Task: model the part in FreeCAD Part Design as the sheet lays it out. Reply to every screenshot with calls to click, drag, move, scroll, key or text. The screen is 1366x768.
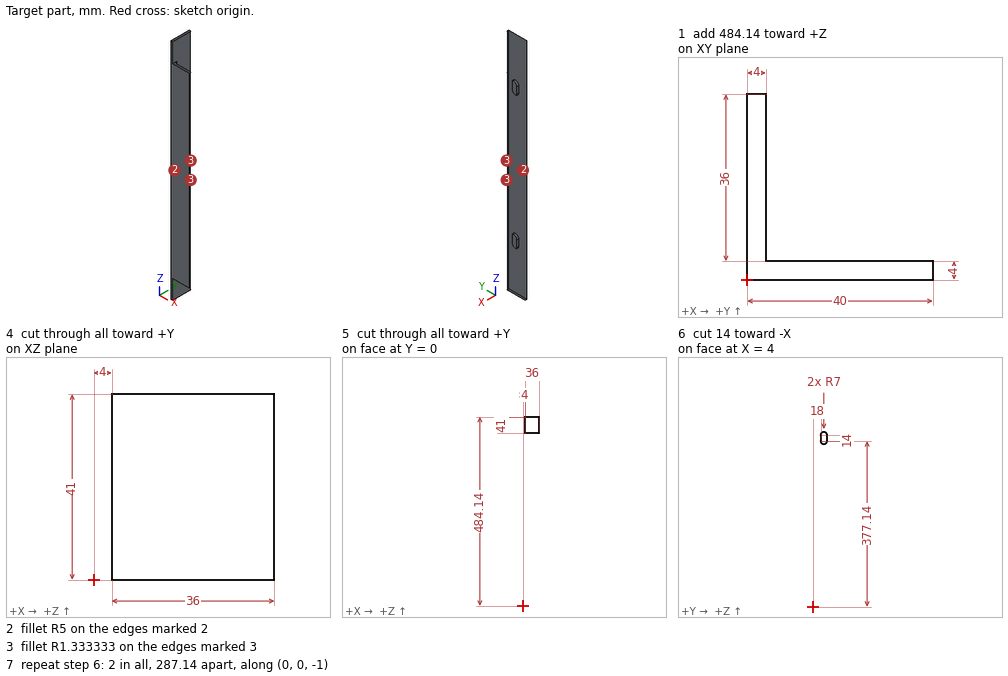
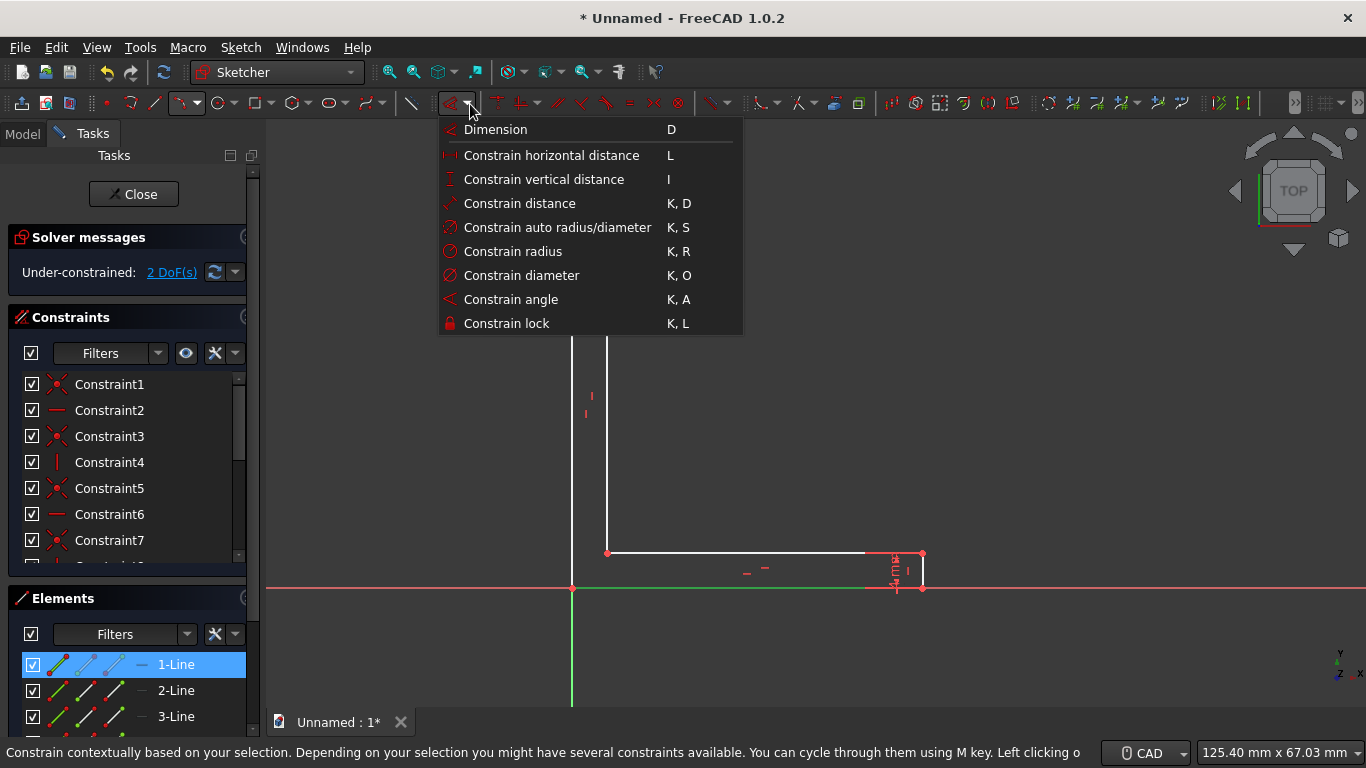
click(591, 155)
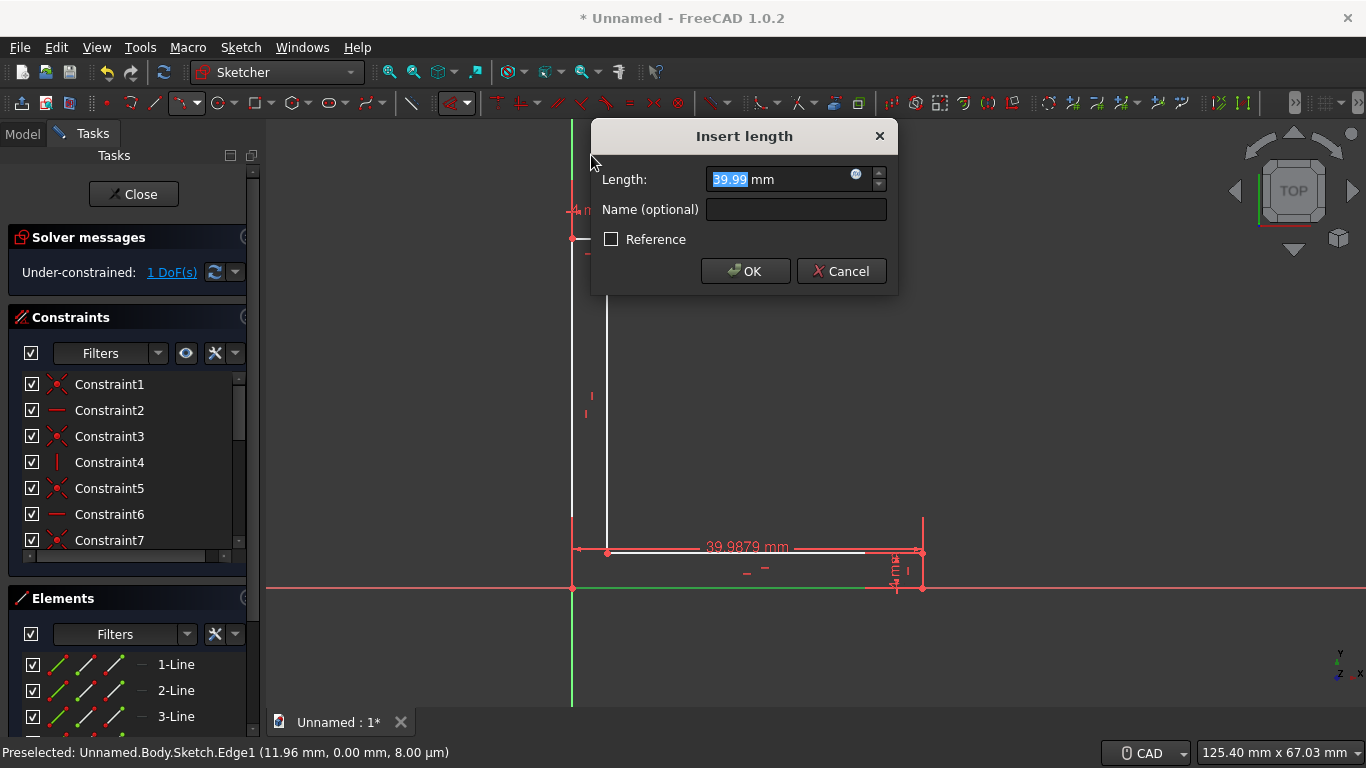
text(40)
key(Return)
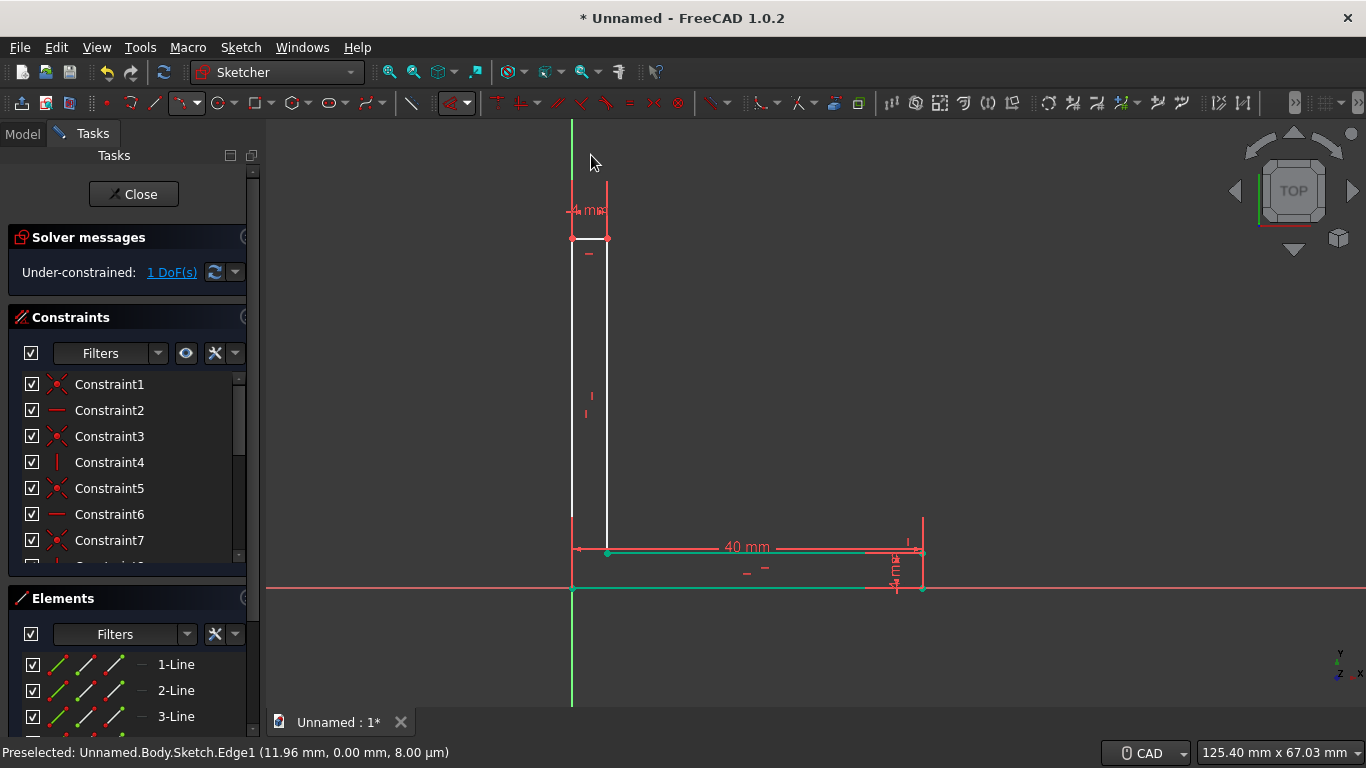
click(607, 459)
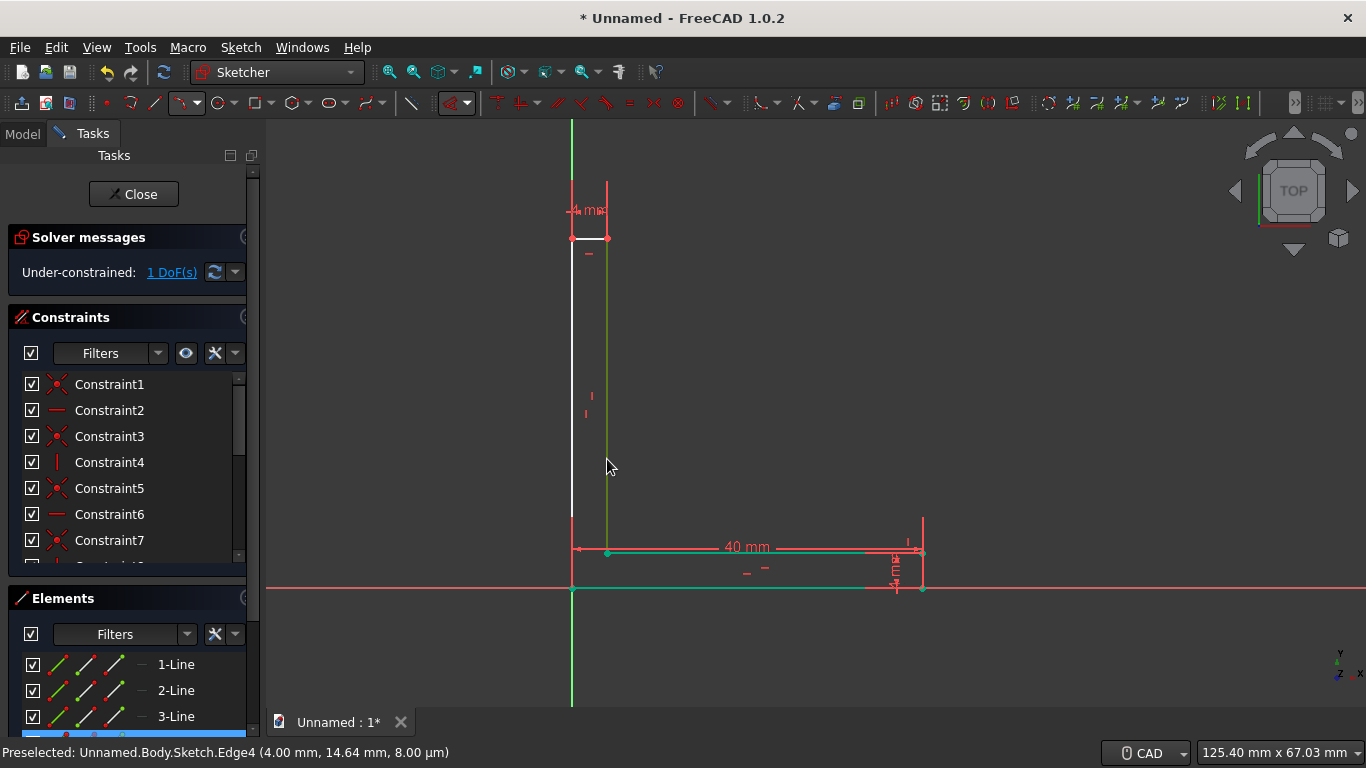
click(470, 104)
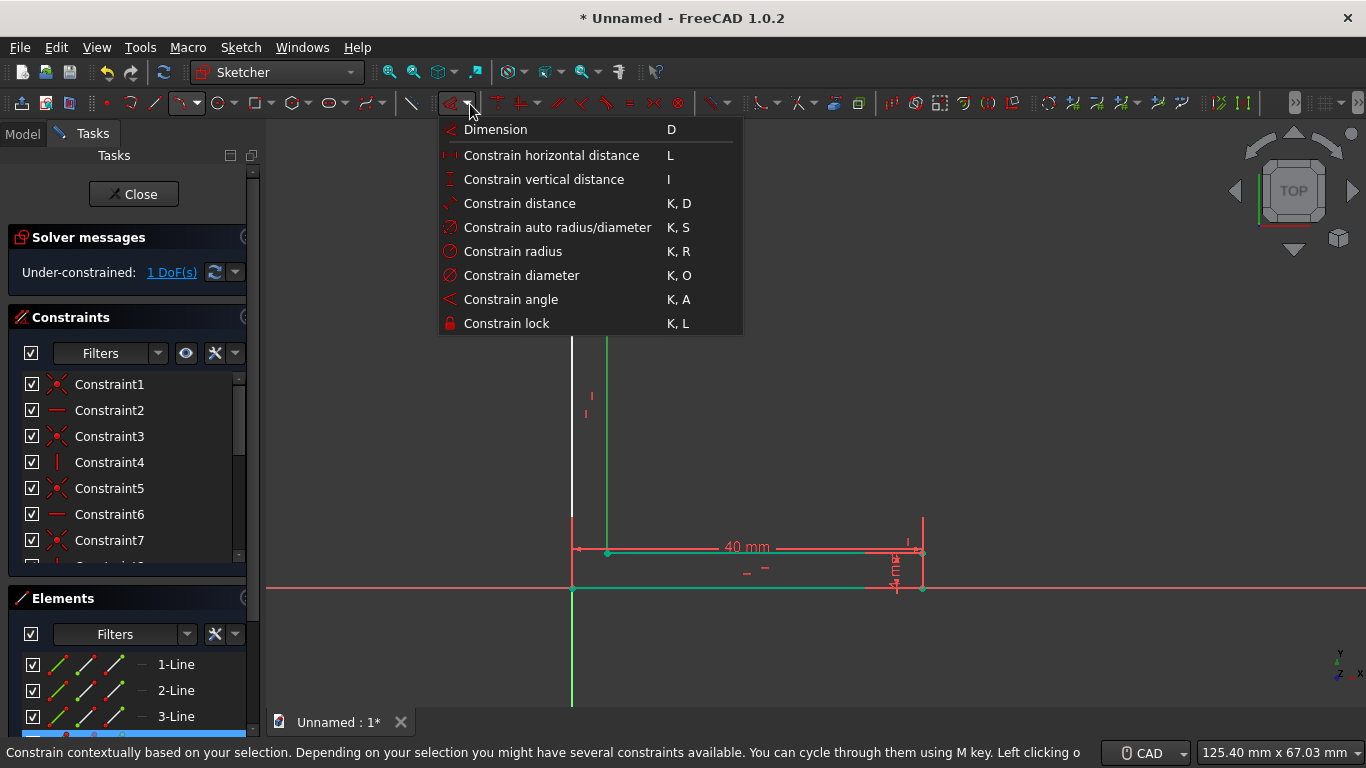
click(591, 179)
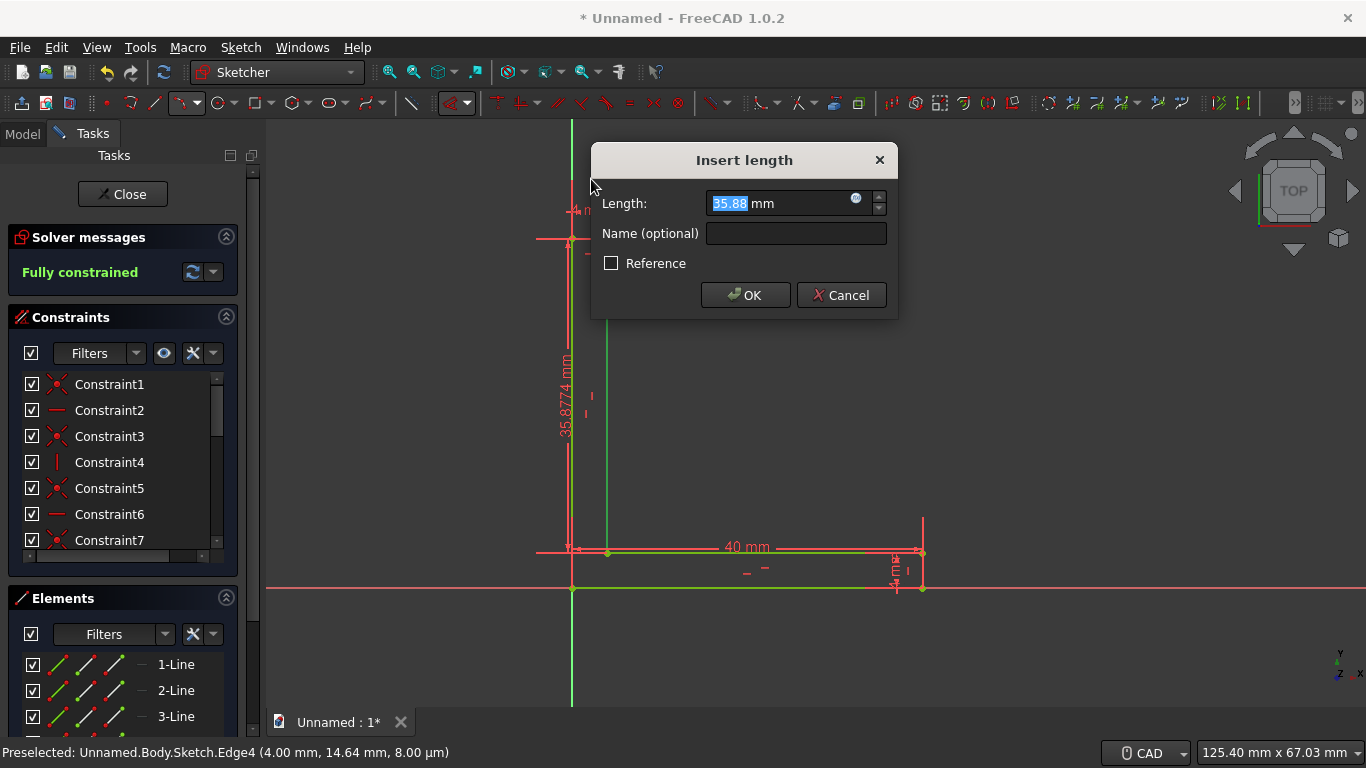
text(36)
key(Return)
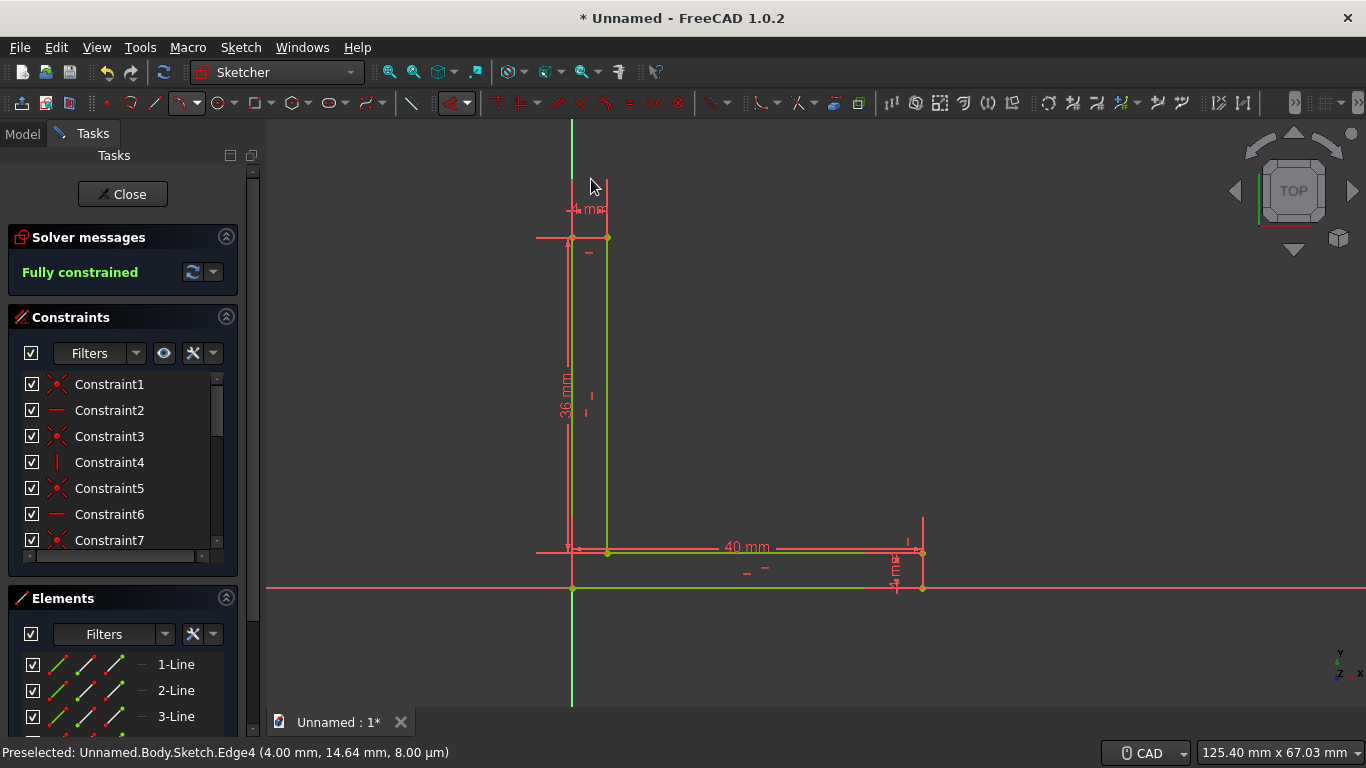
click(123, 194)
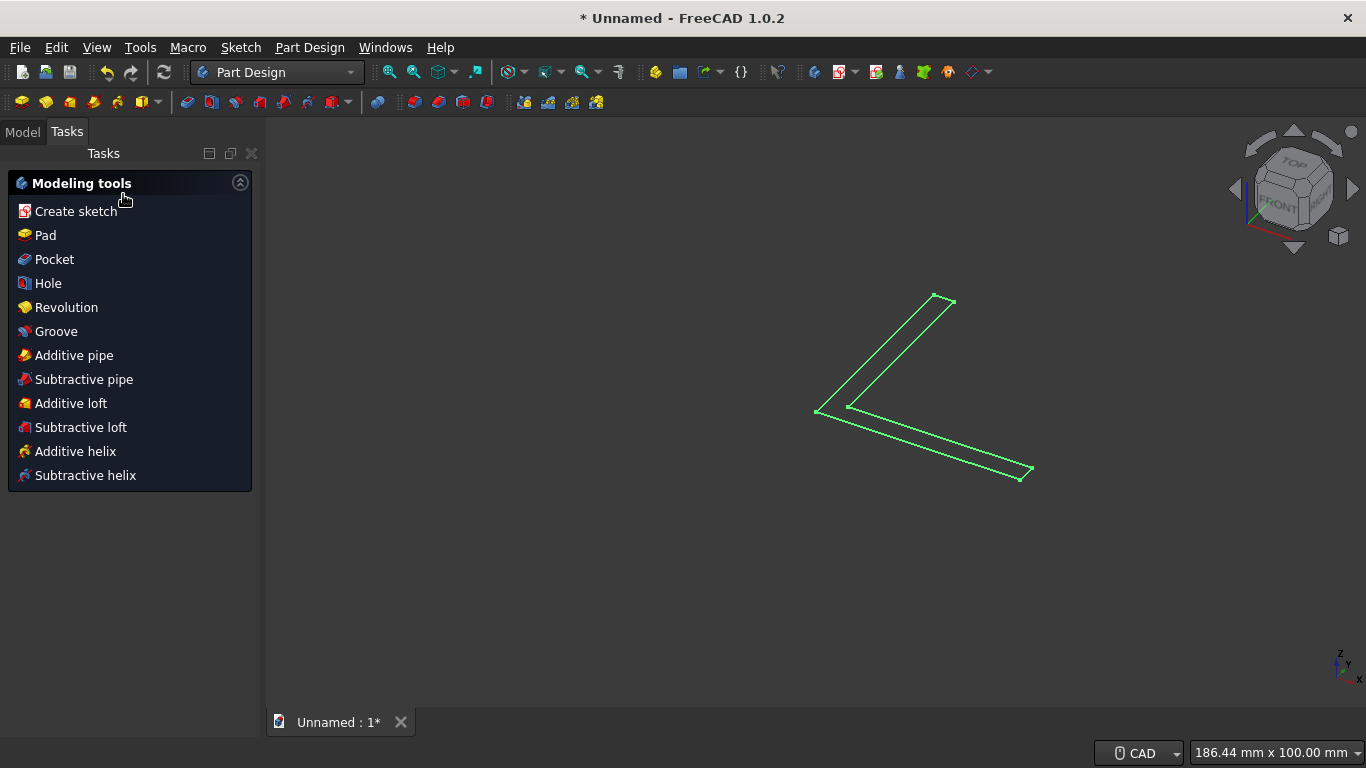
click(22, 102)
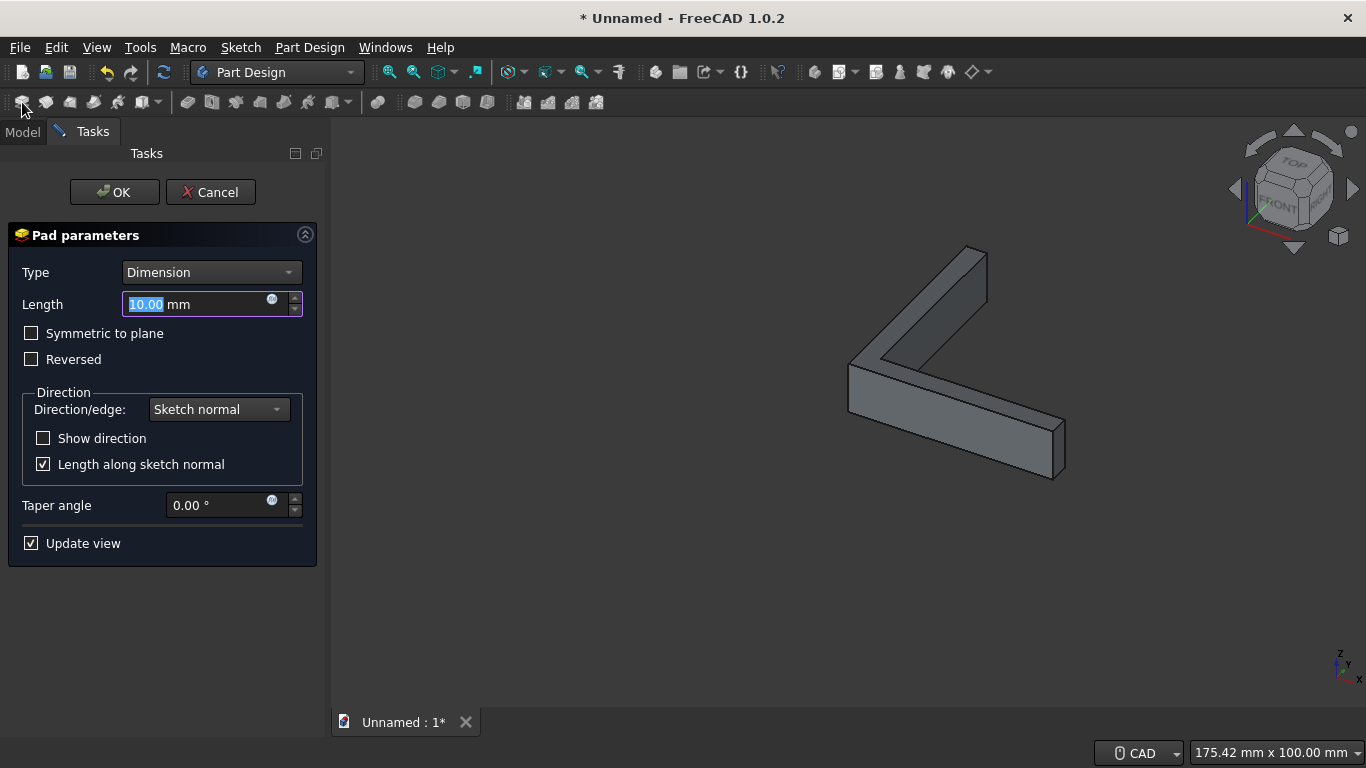
text(484.14)
key(Tab)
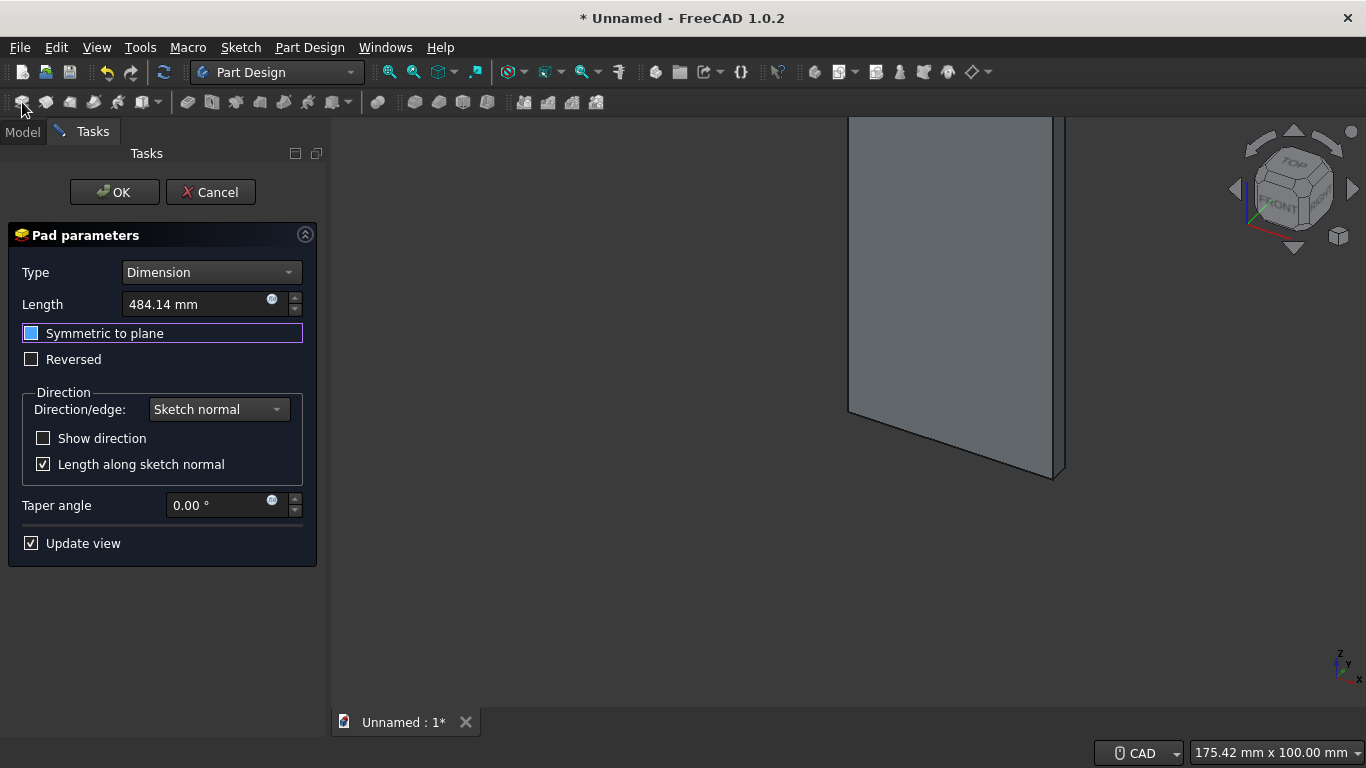
click(115, 192)